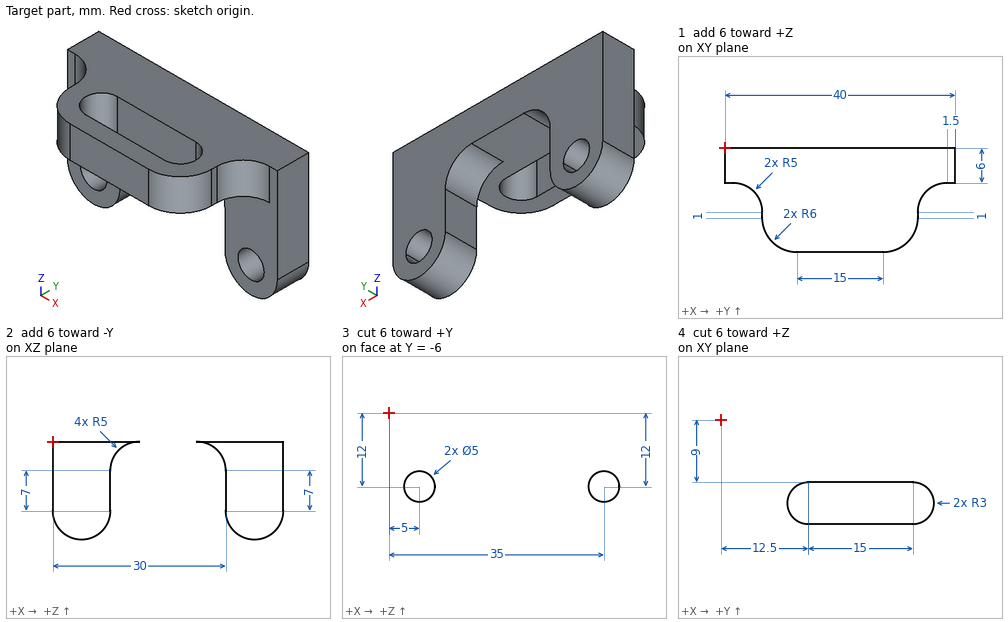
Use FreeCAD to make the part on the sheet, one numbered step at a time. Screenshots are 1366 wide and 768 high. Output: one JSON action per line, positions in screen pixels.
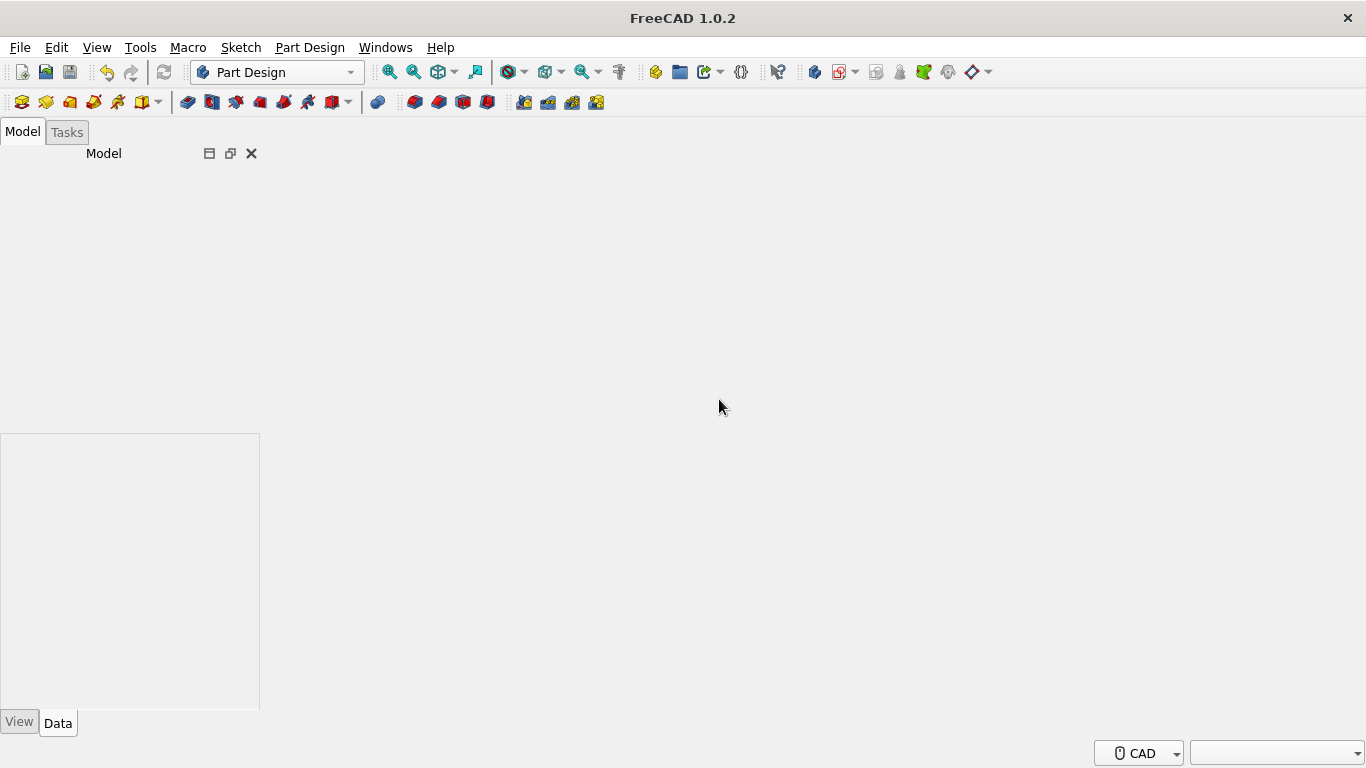
{"action": "key", "text": "ctrl+n"}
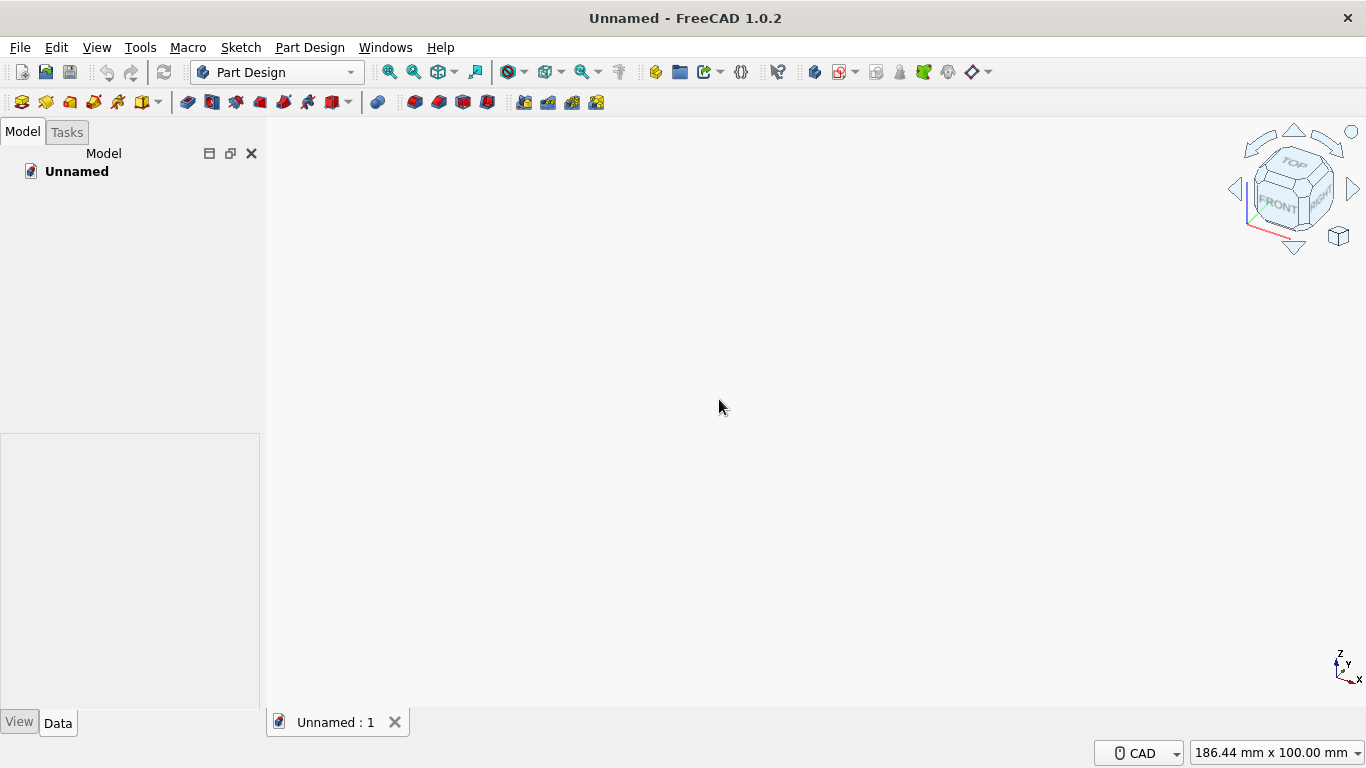
{"action": "left_click", "coordinate": [840, 72]}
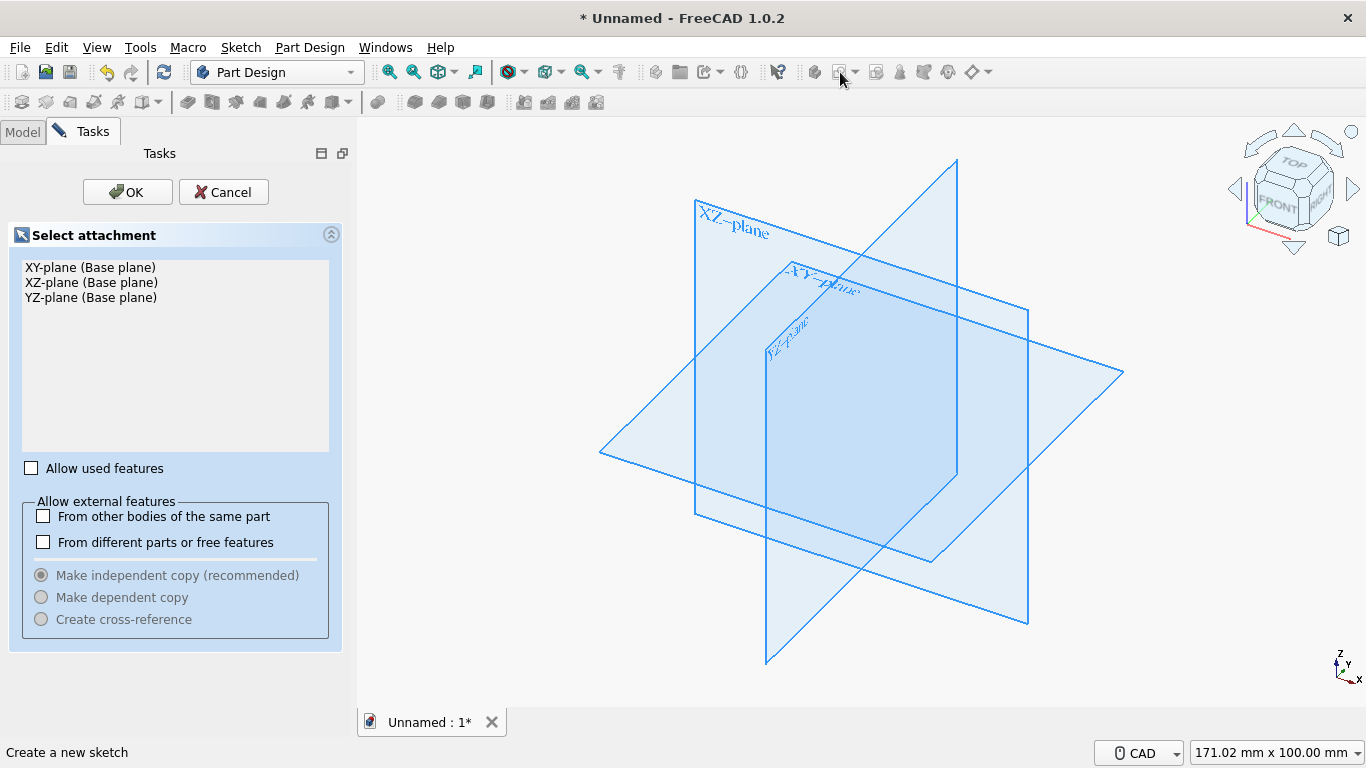
{"action": "left_click", "coordinate": [82, 268]}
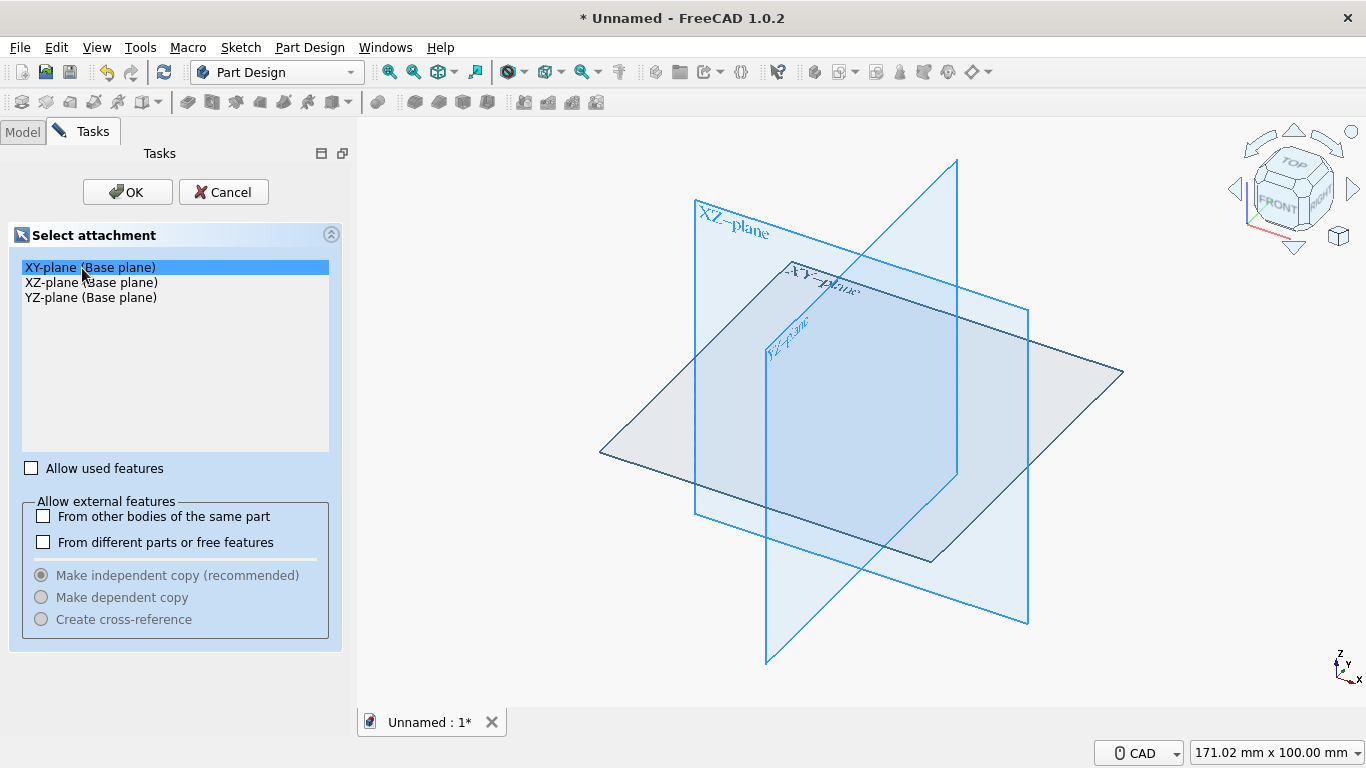
{"action": "left_click", "coordinate": [128, 192]}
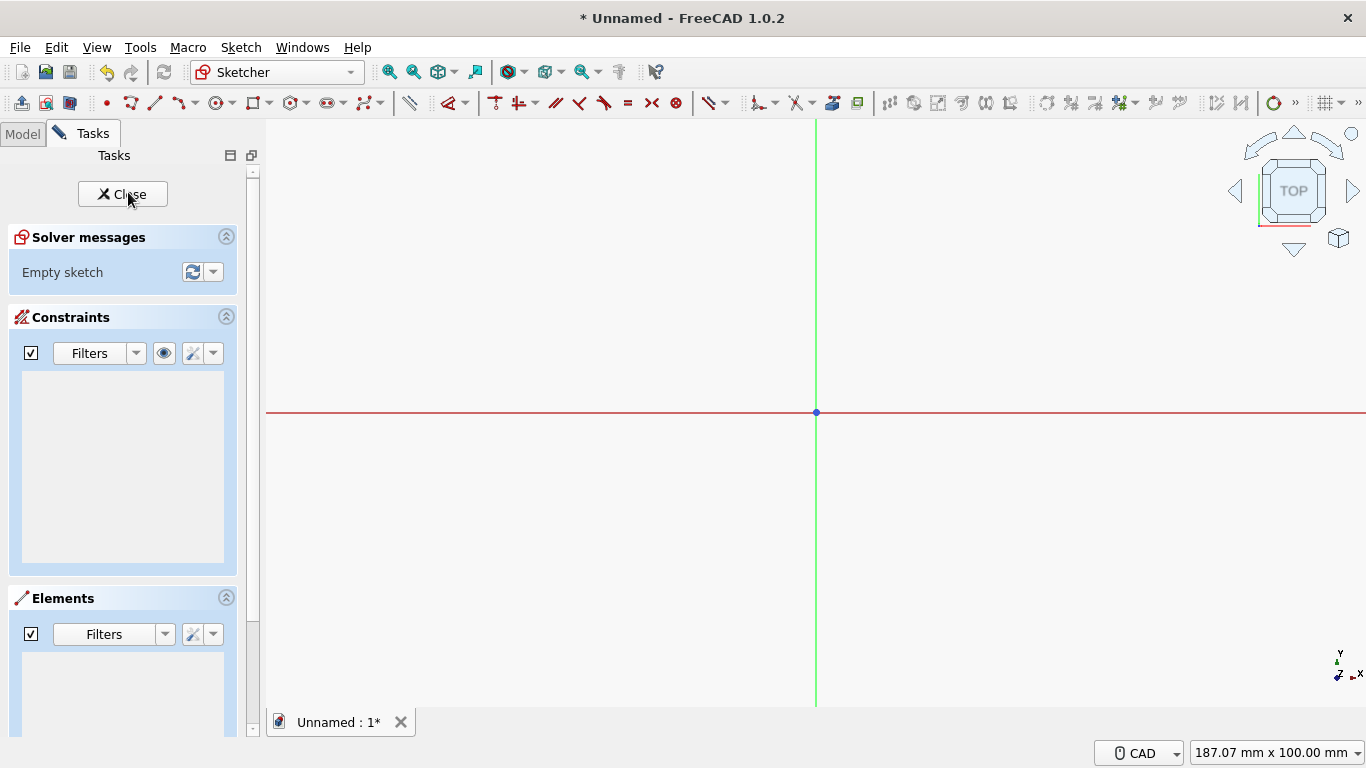
{"action": "scroll", "coordinate": [1042, 497], "scroll_direction": "up", "scroll_amount": 5}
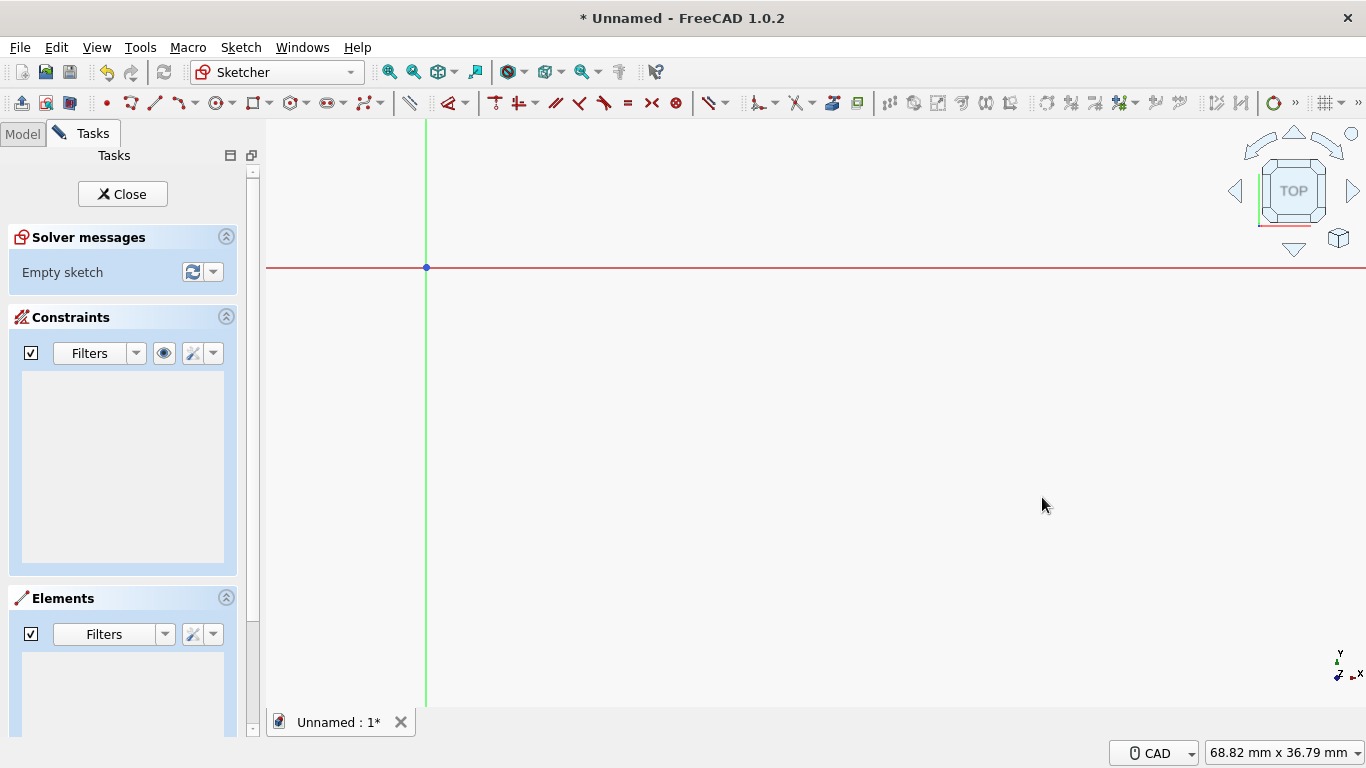
{"action": "key", "text": "g l"}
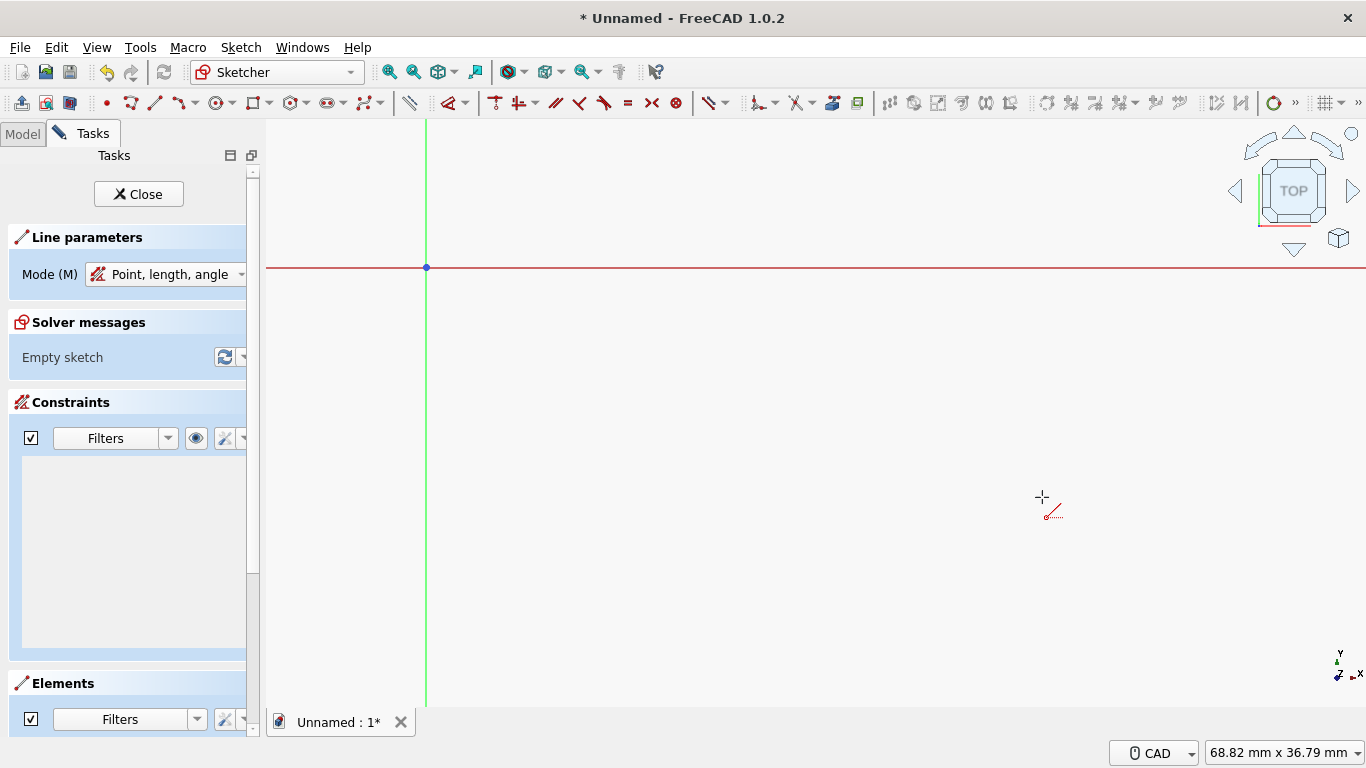
{"action": "left_click", "coordinate": [530, 443]}
{"action": "left_click", "coordinate": [530, 459]}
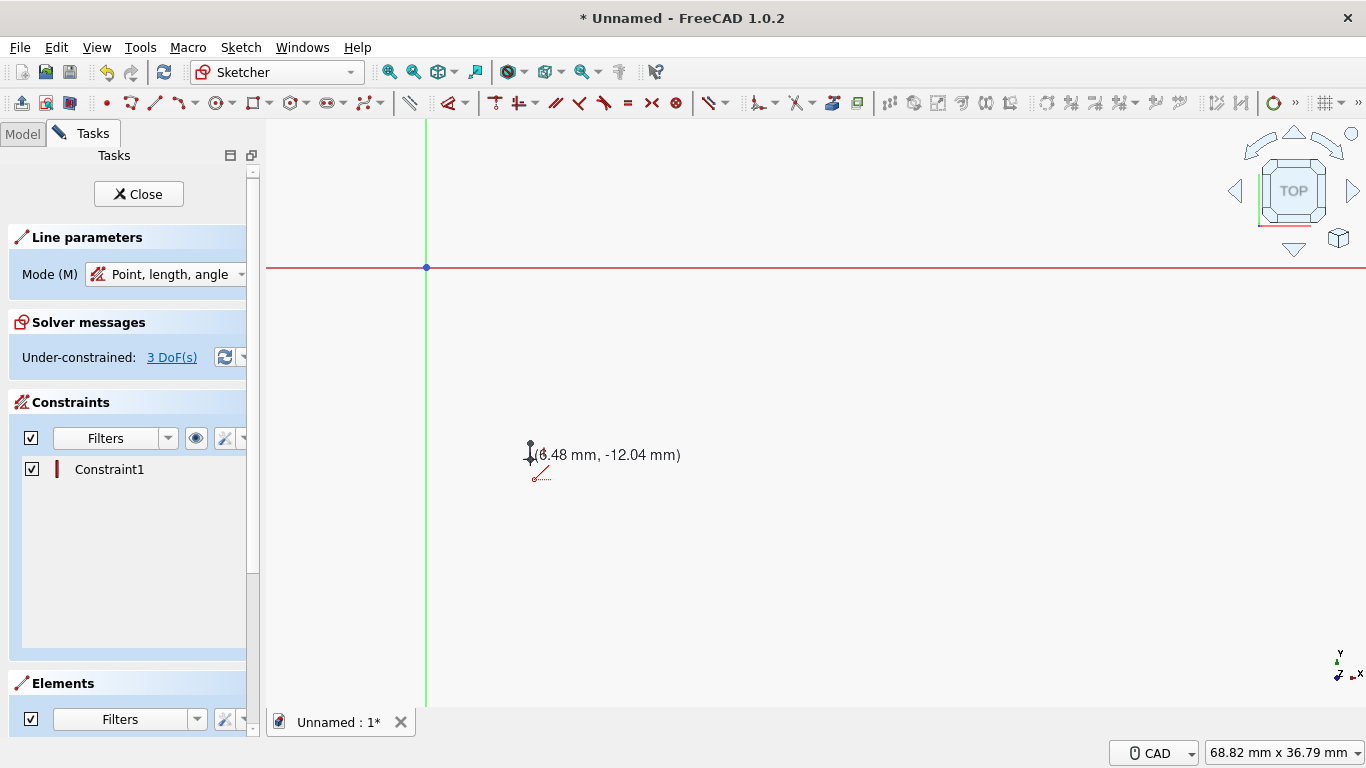
{"action": "left_click", "coordinate": [626, 555]}
{"action": "left_click", "coordinate": [866, 555]}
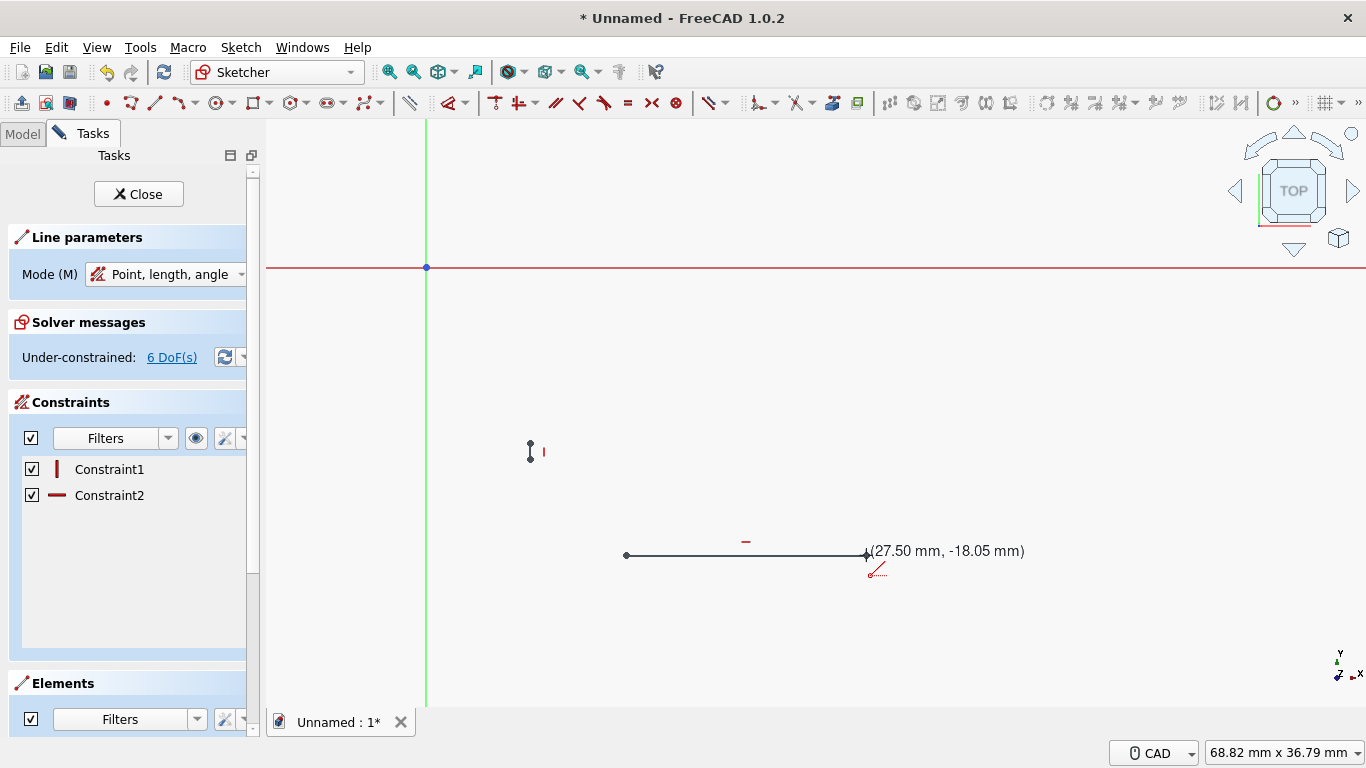
{"action": "left_click", "coordinate": [962, 459]}
{"action": "left_click", "coordinate": [962, 443]}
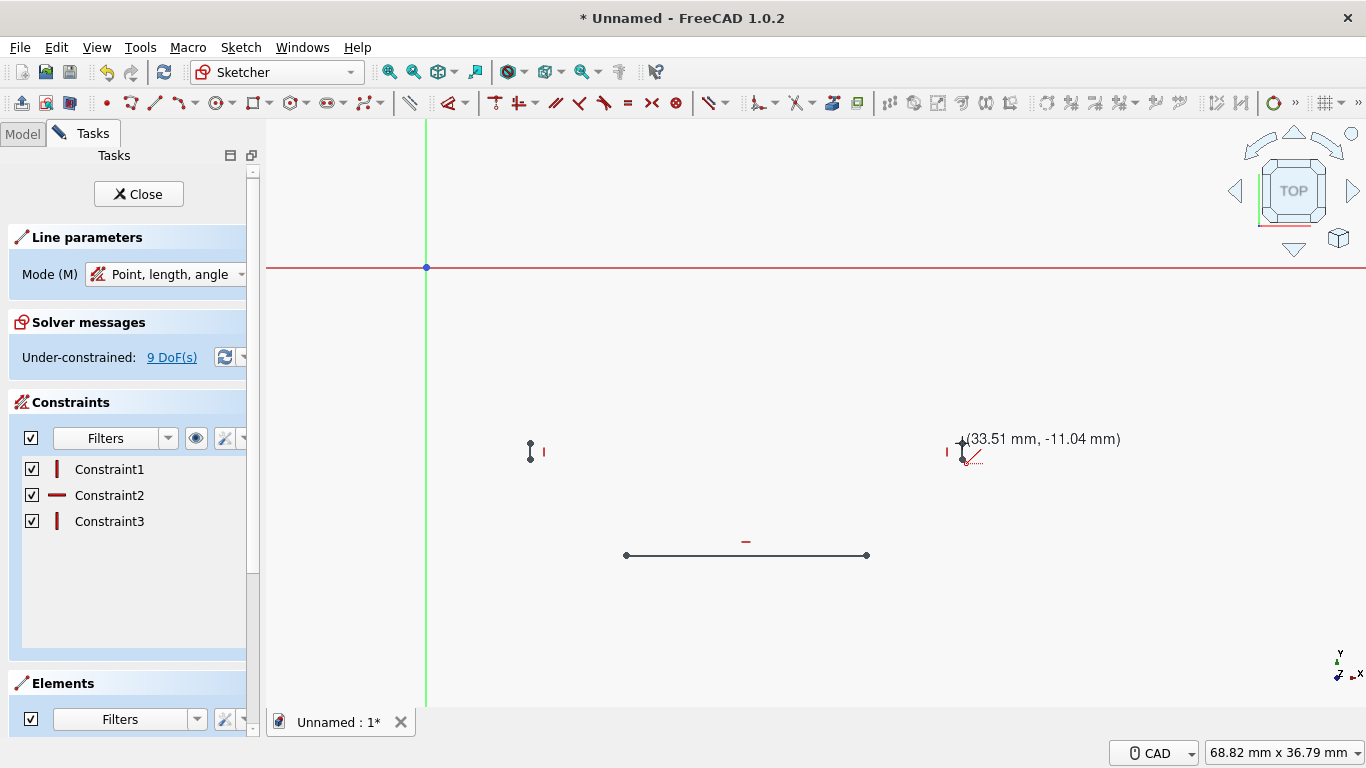
{"action": "key", "text": "g m"}